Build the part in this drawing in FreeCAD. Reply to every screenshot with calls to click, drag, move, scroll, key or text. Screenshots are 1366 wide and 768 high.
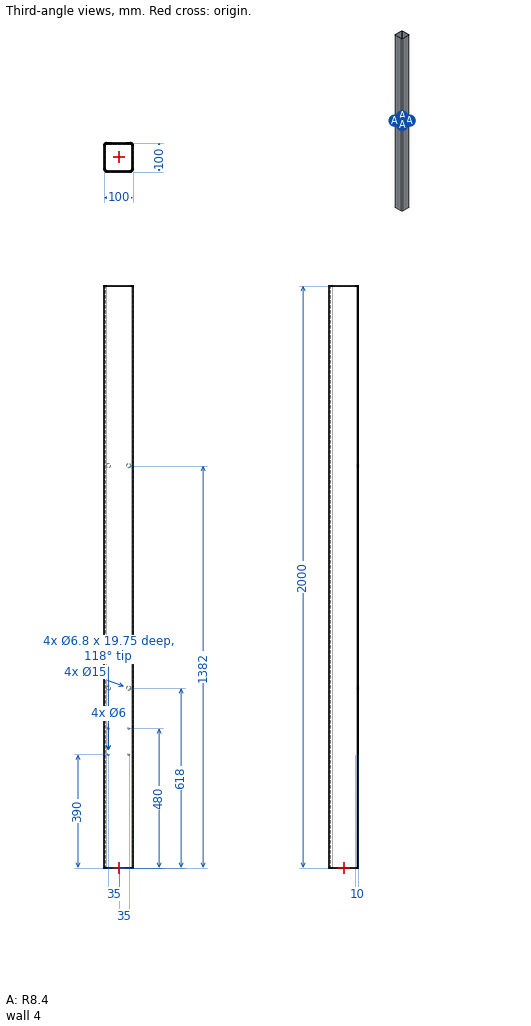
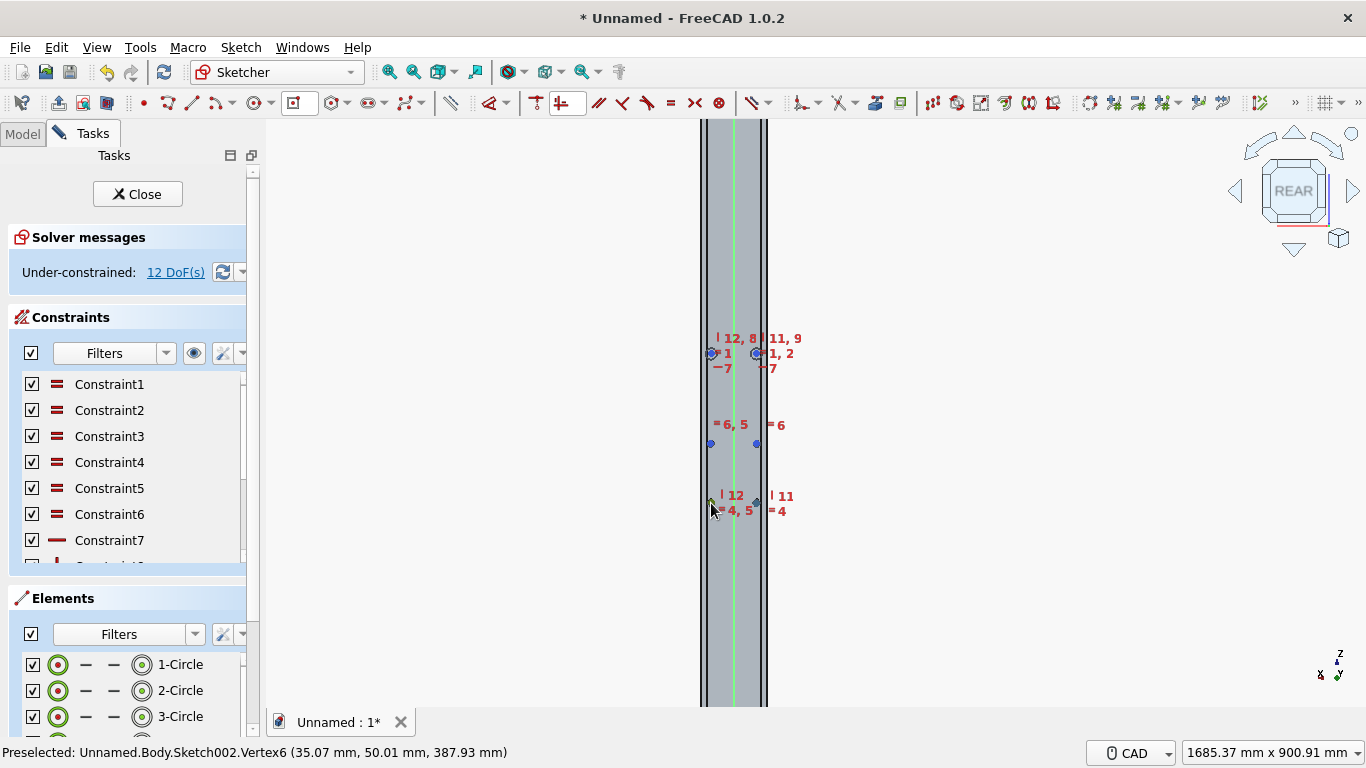
key(h)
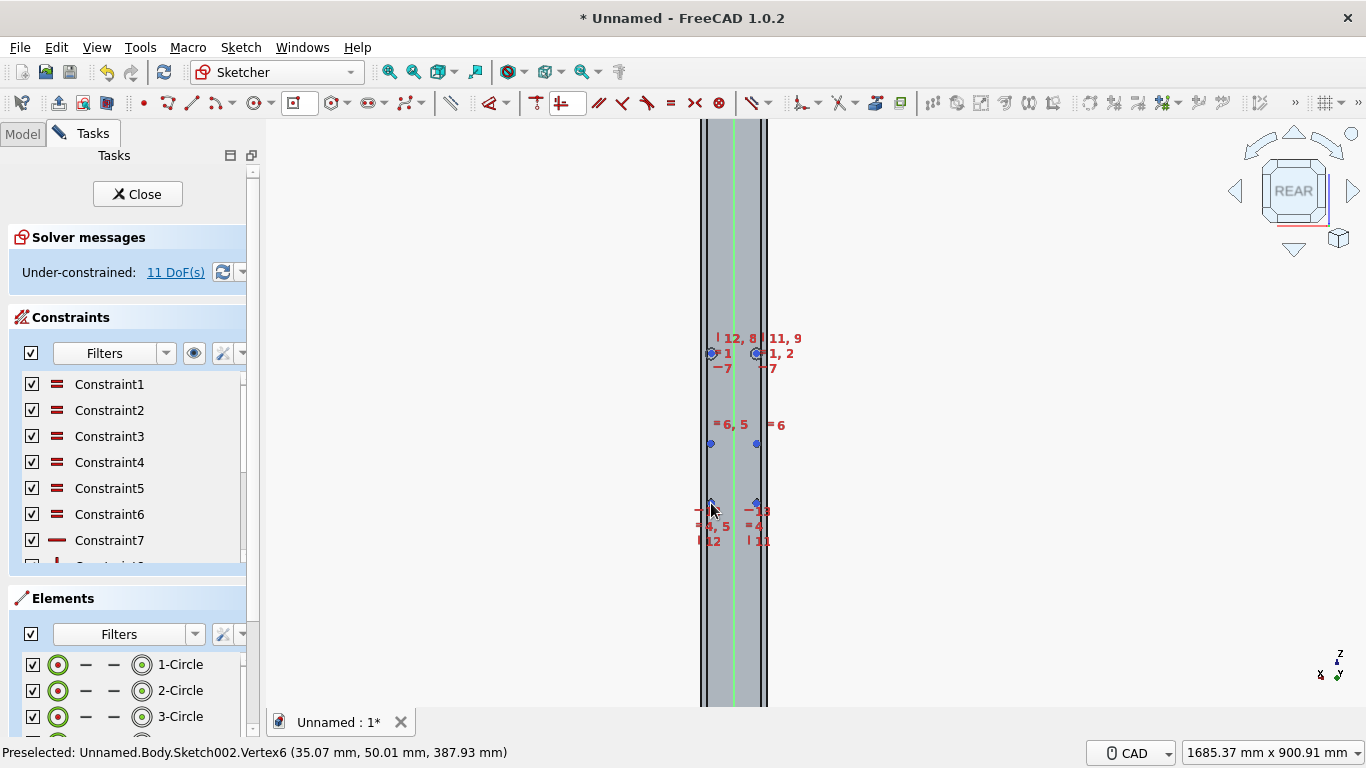
click(711, 503)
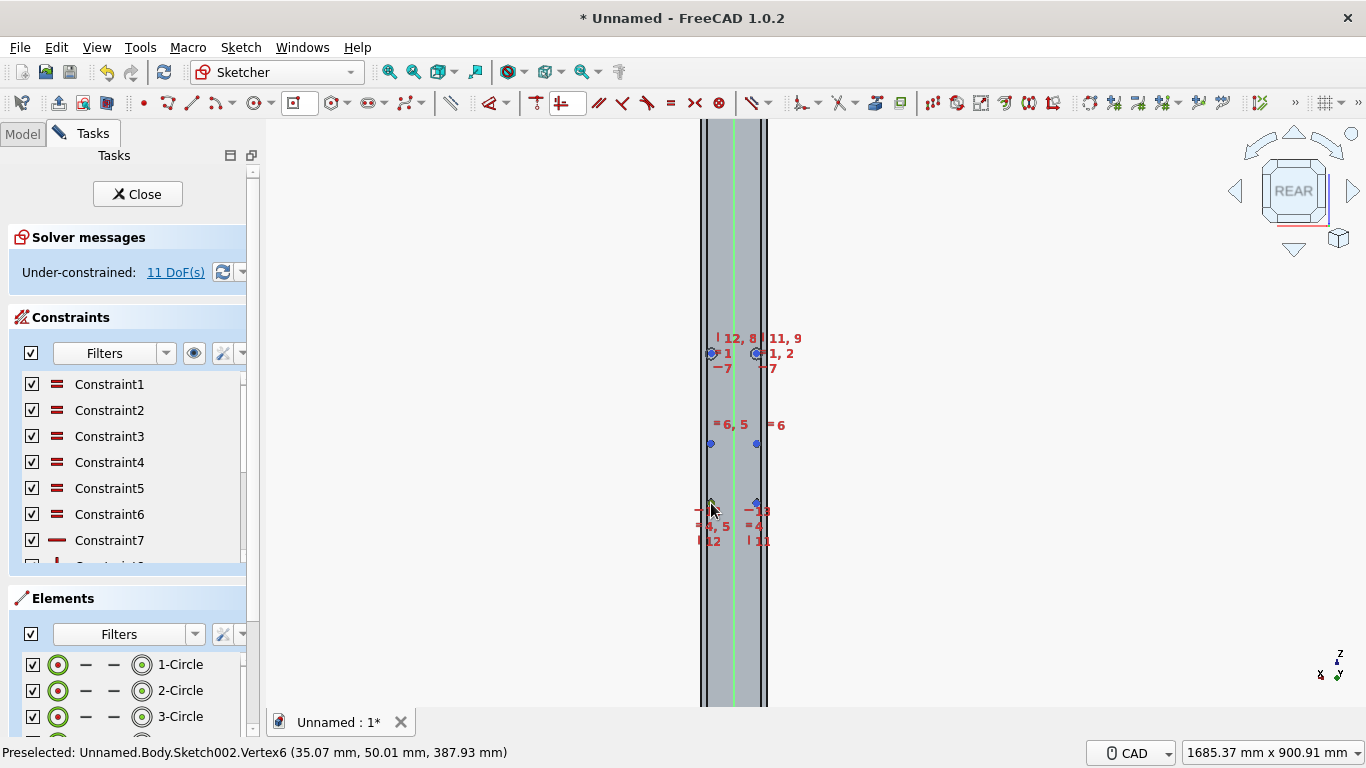
click(711, 444)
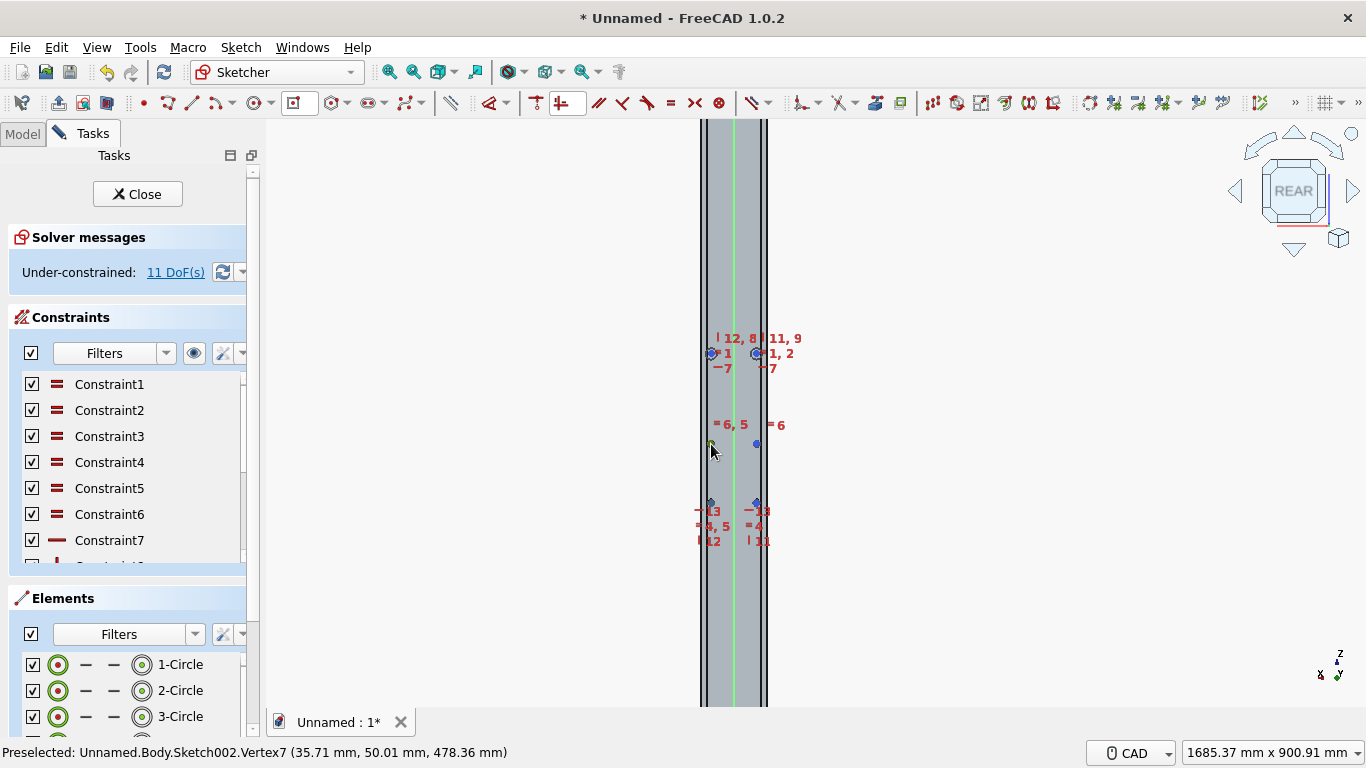
key(v)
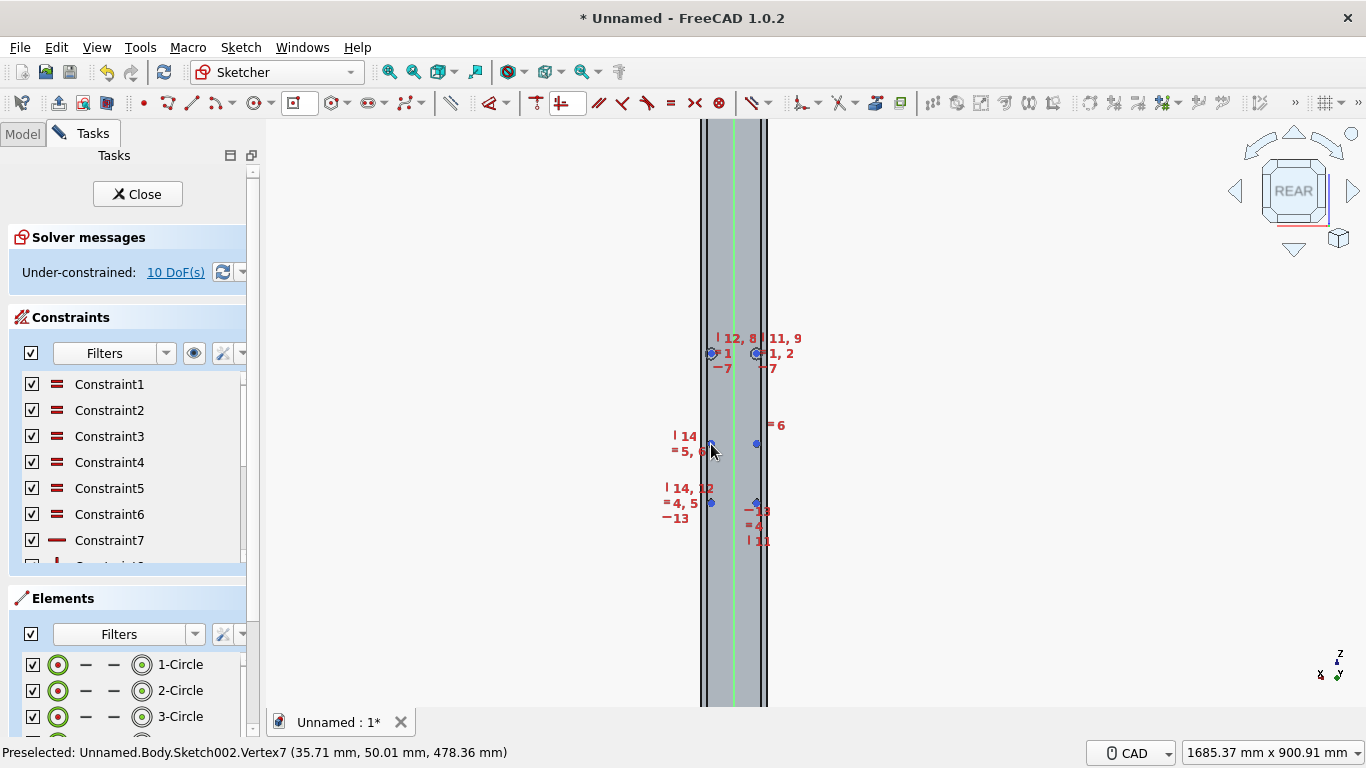
click(756, 503)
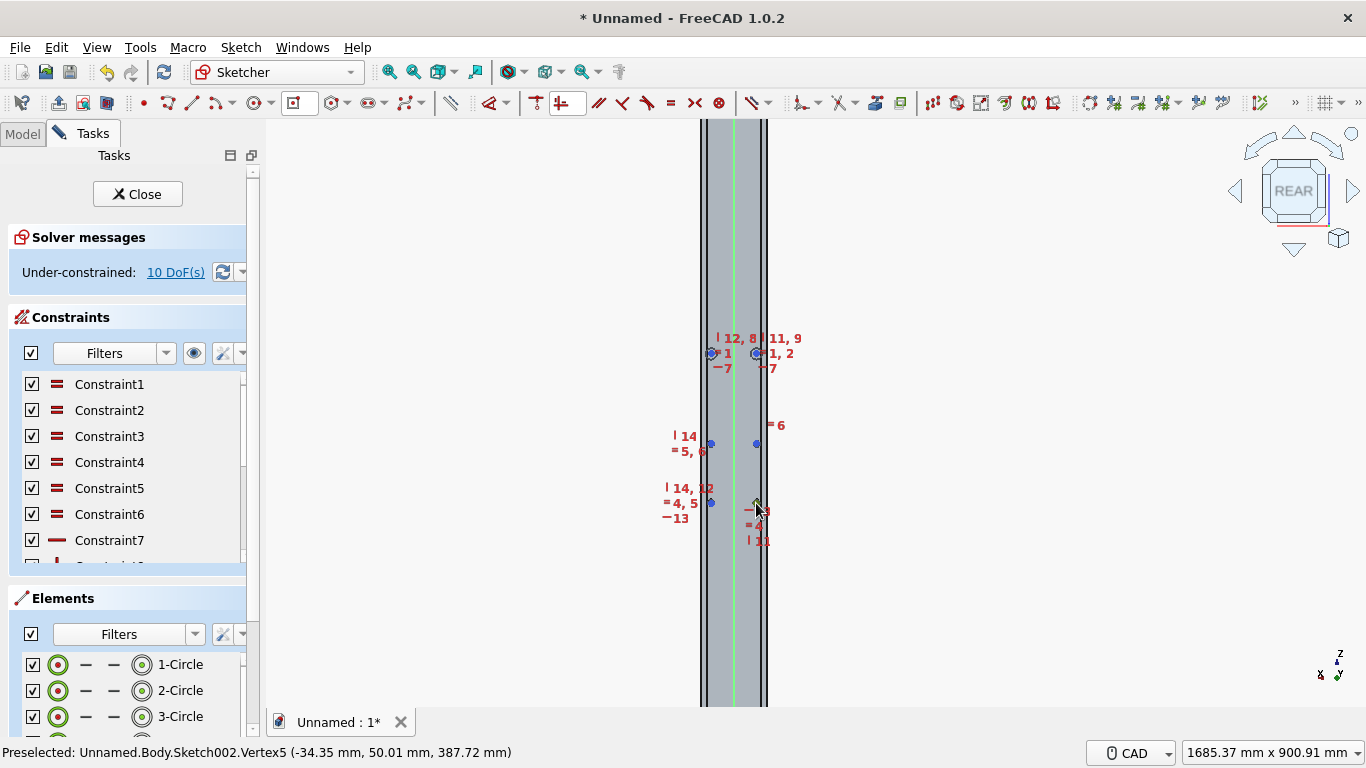
click(757, 444)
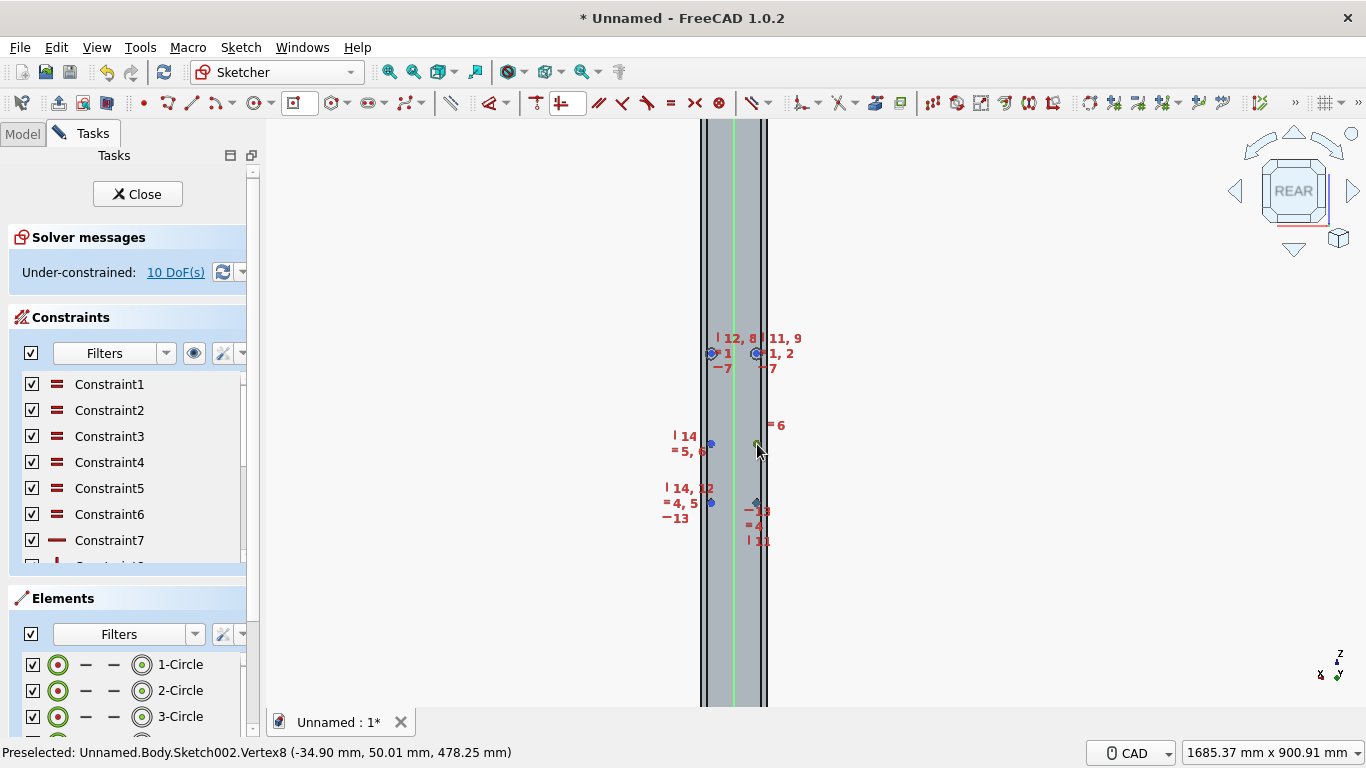
key(v)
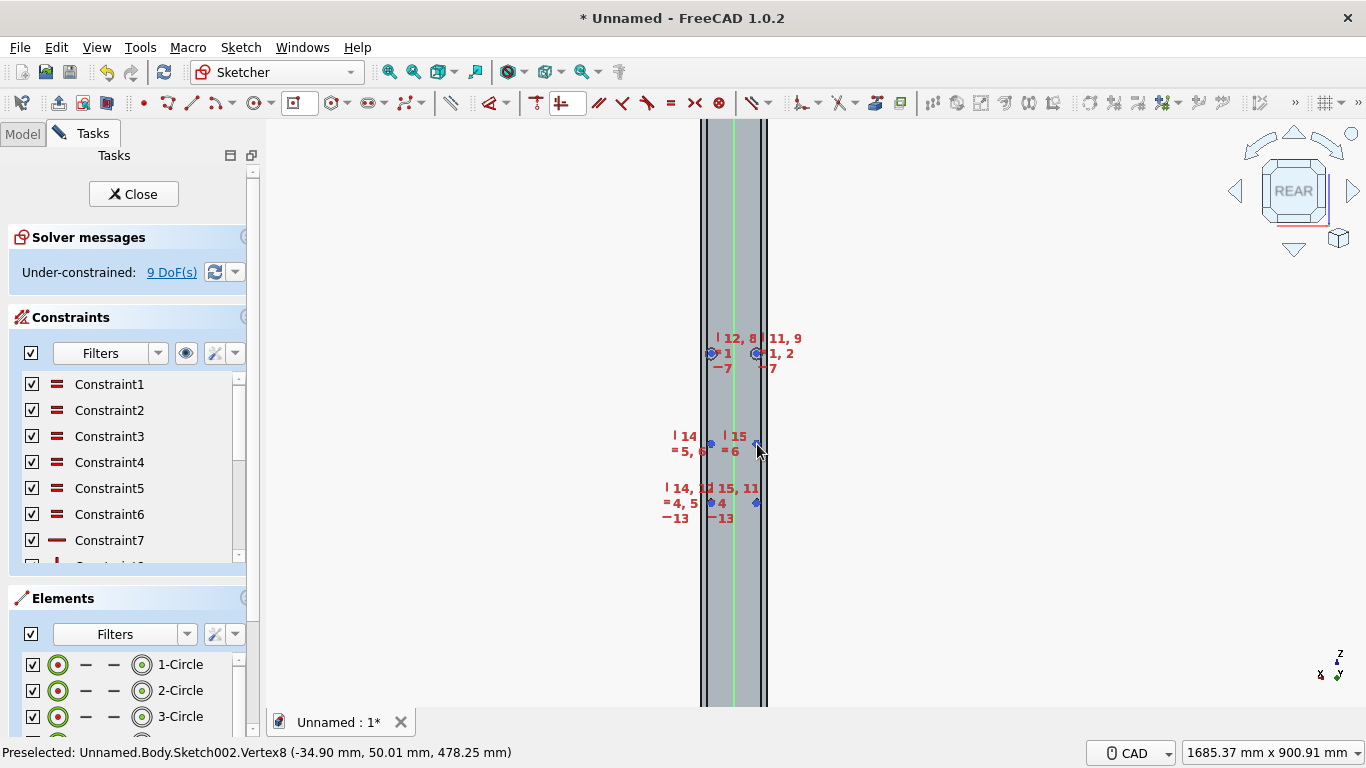
click(711, 444)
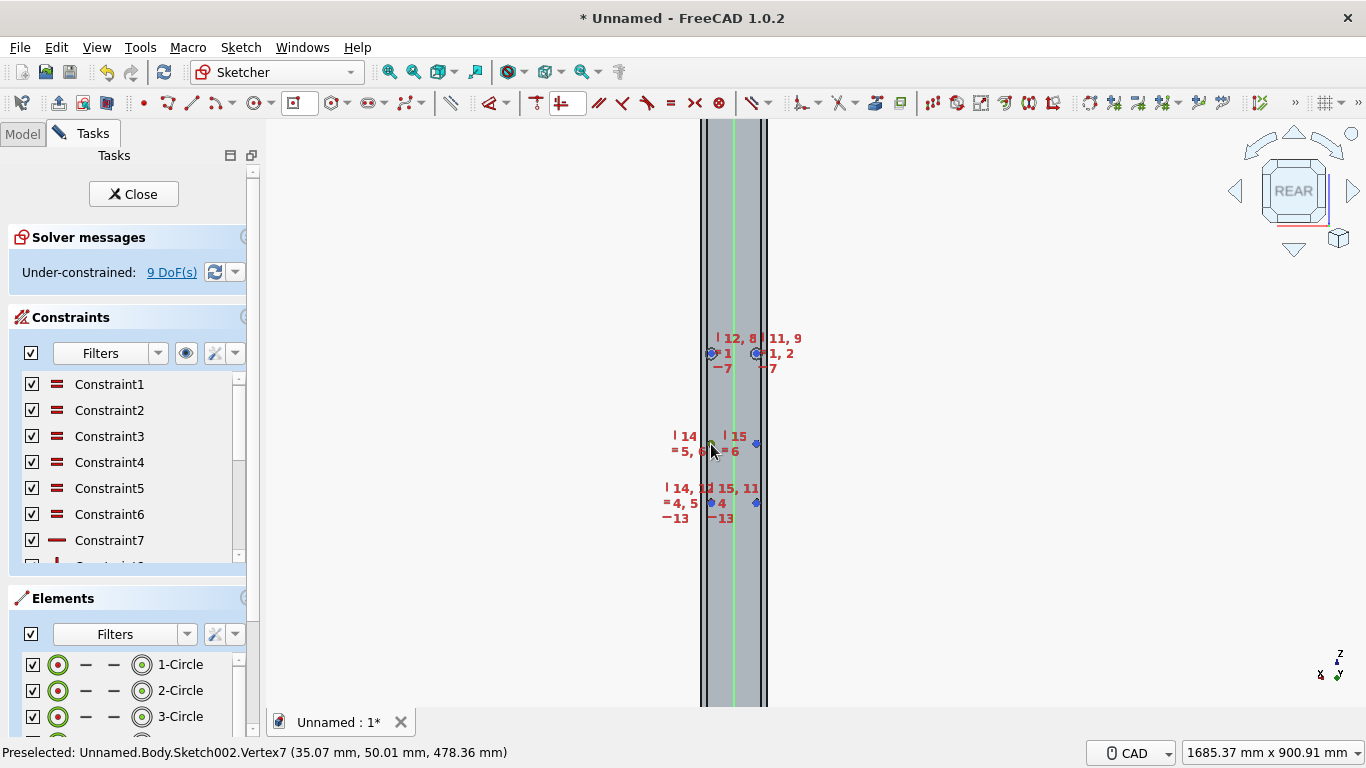
click(756, 444)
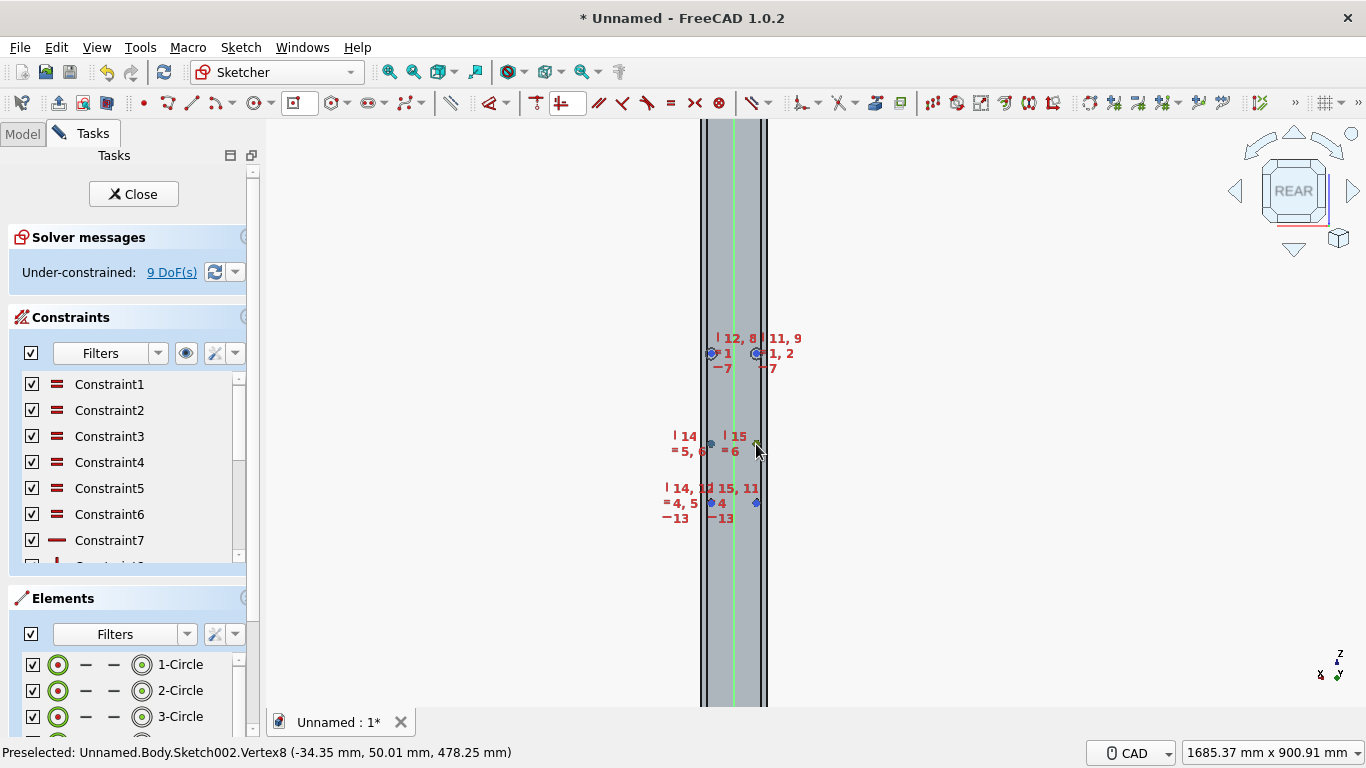
click(580, 104)